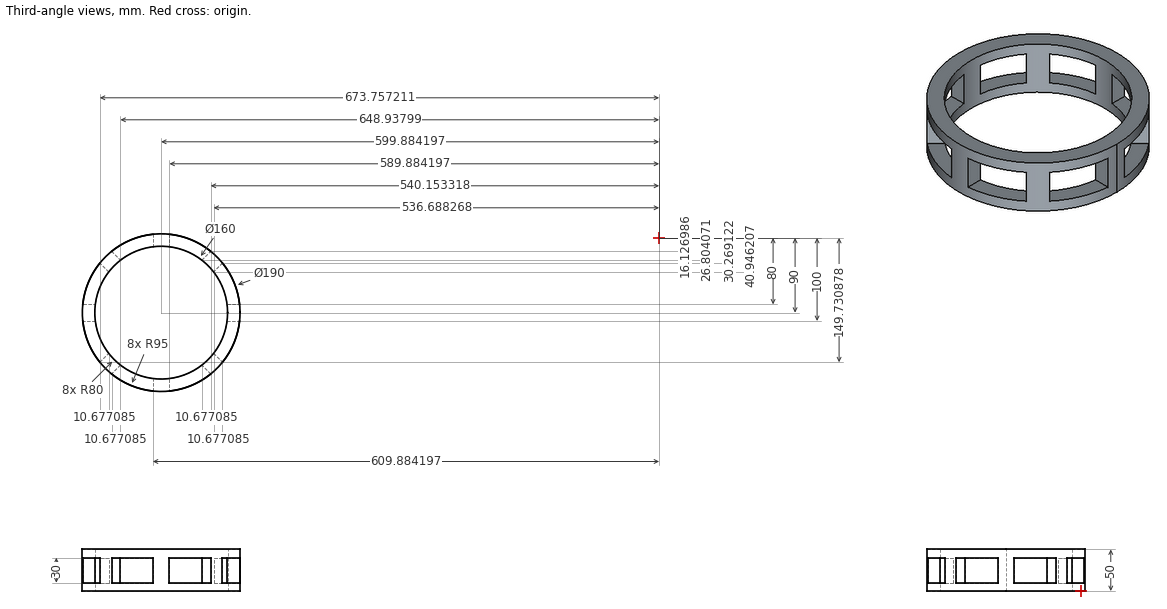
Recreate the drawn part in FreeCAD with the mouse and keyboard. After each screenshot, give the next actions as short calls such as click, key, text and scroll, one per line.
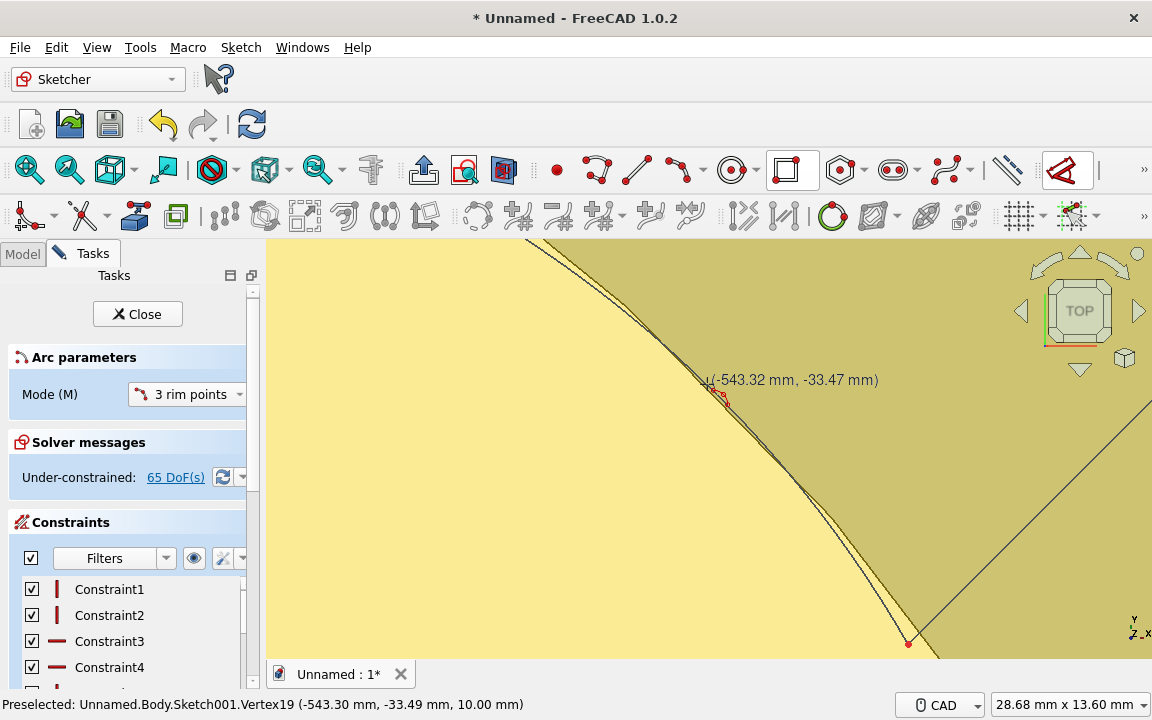
scroll(729, 361, down, 15)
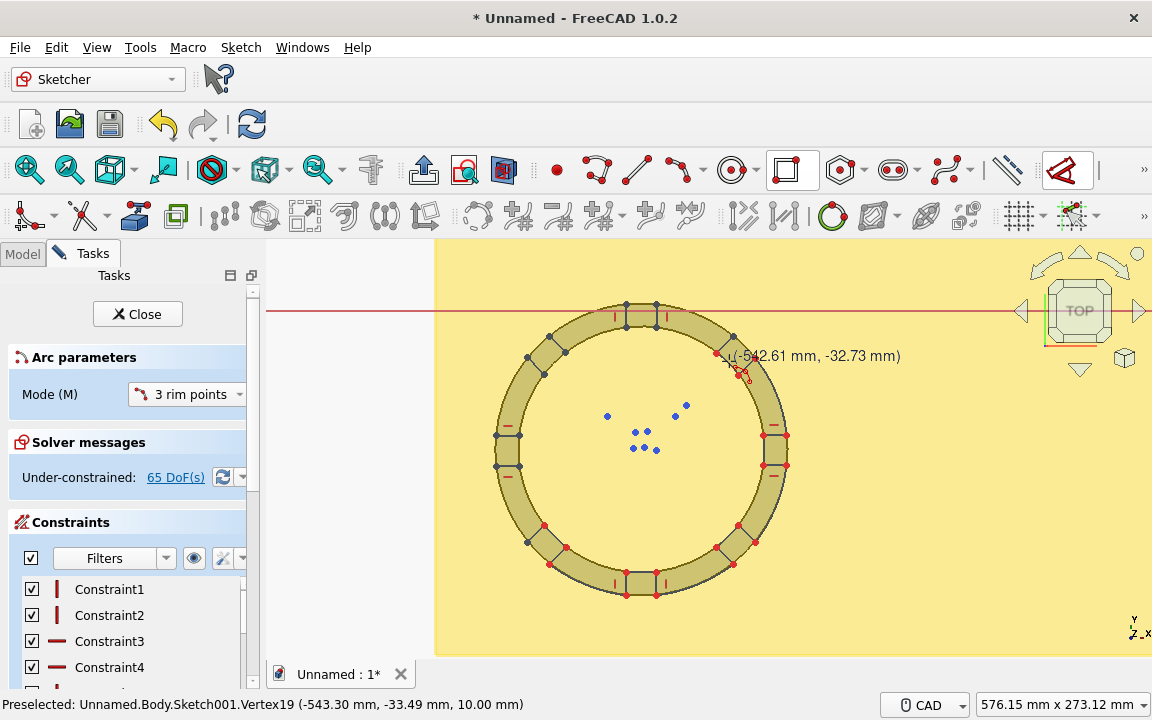
scroll(733, 336, up, 2)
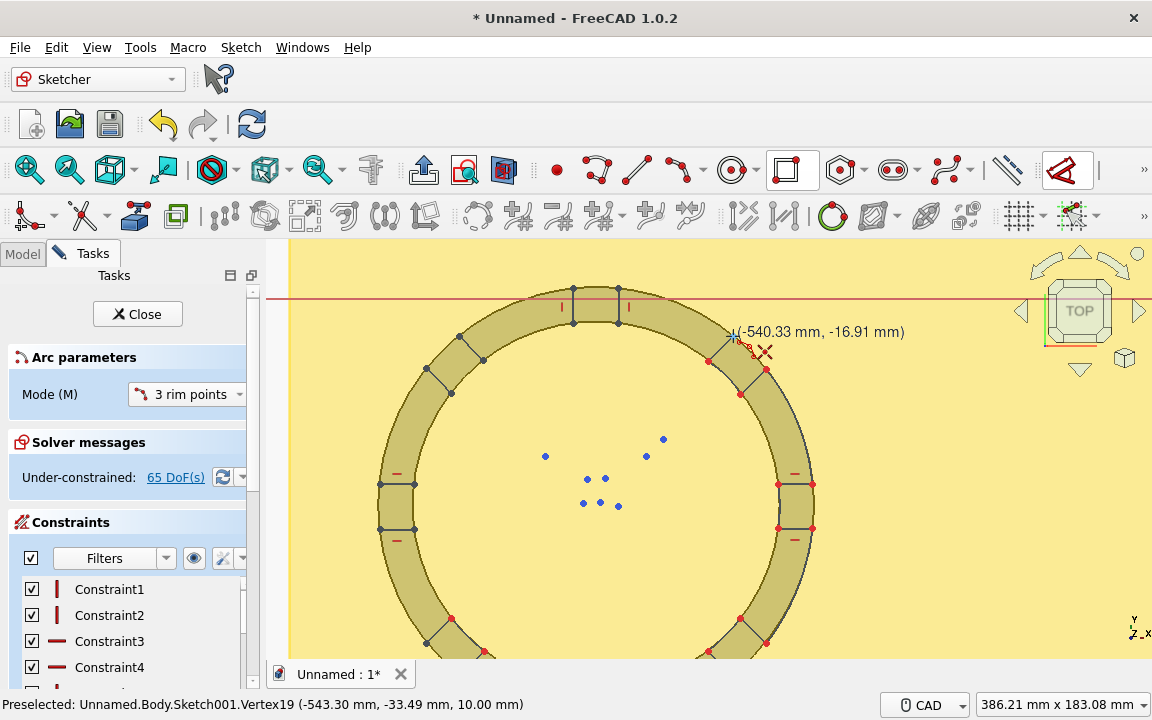
click(733, 336)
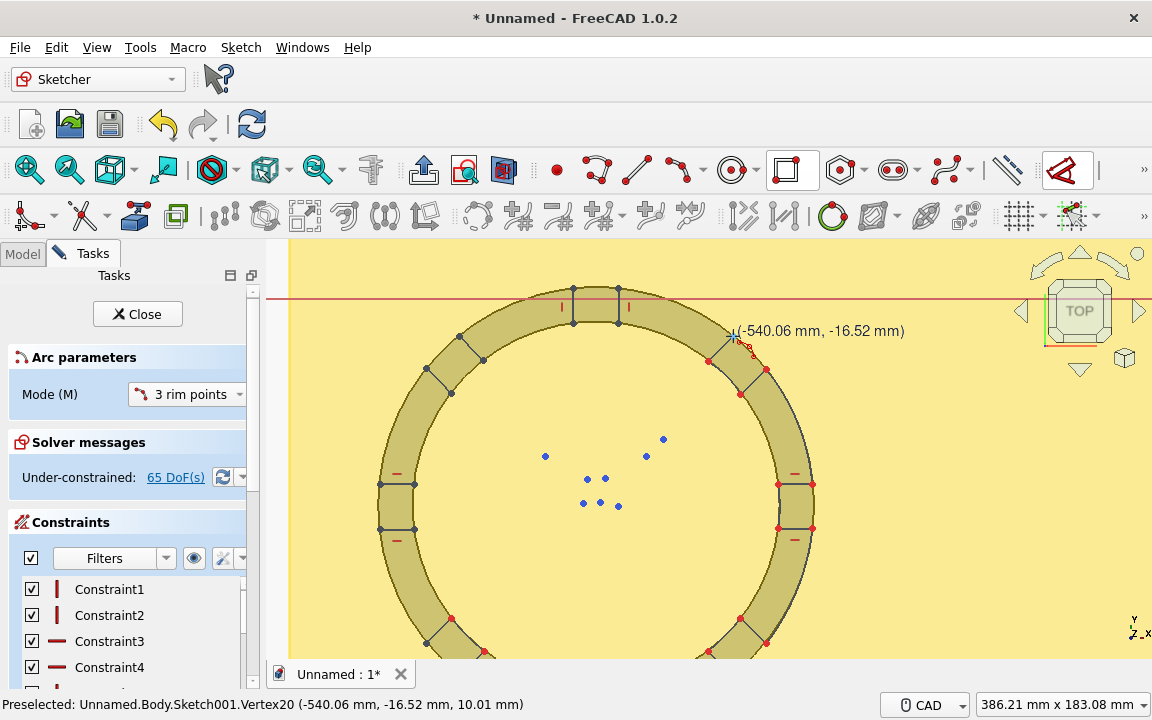
scroll(619, 288, up, 3)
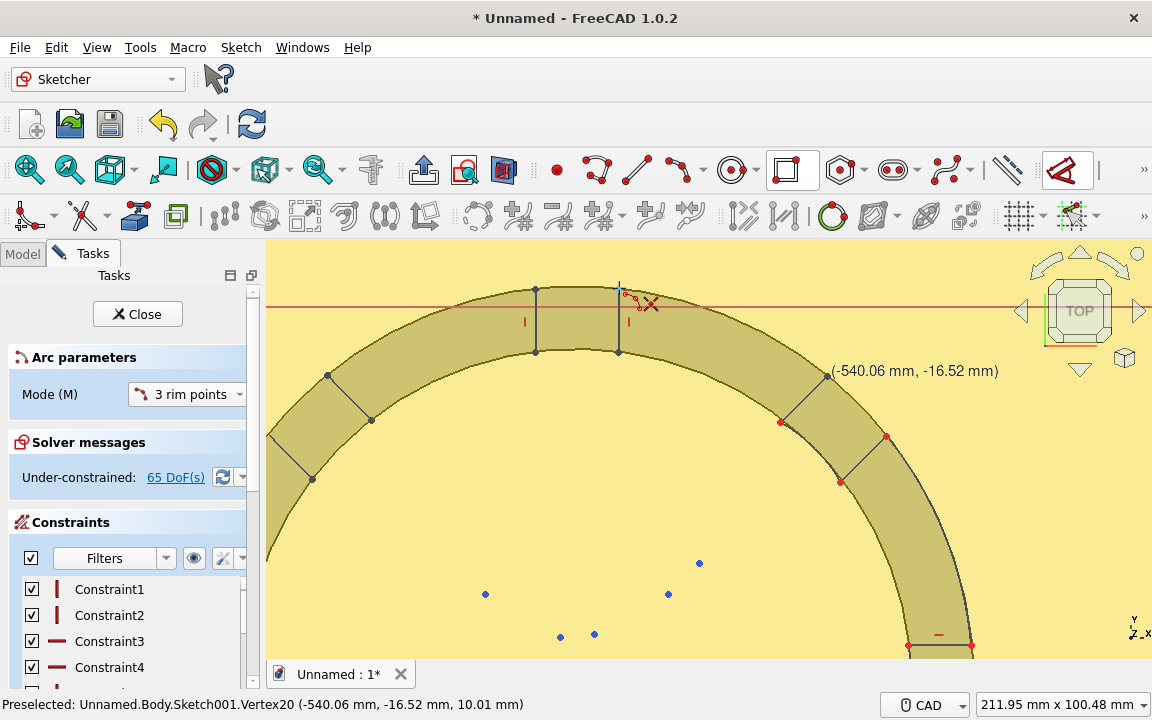
click(619, 290)
click(750, 326)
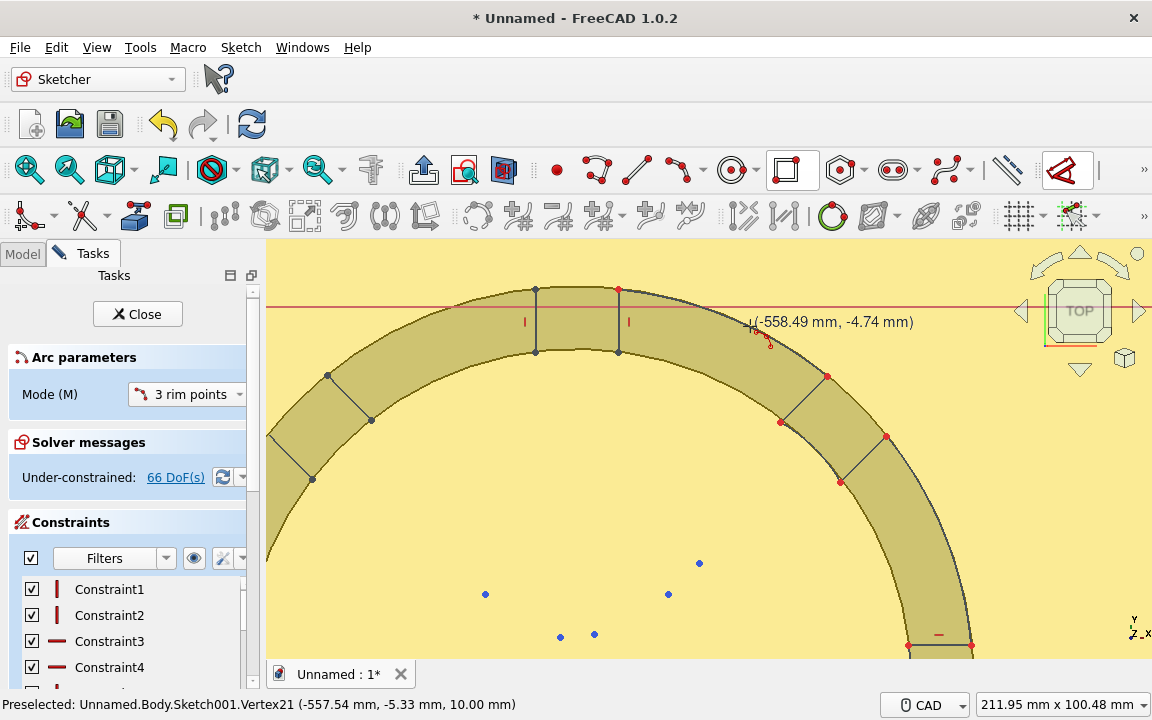
click(619, 353)
click(536, 353)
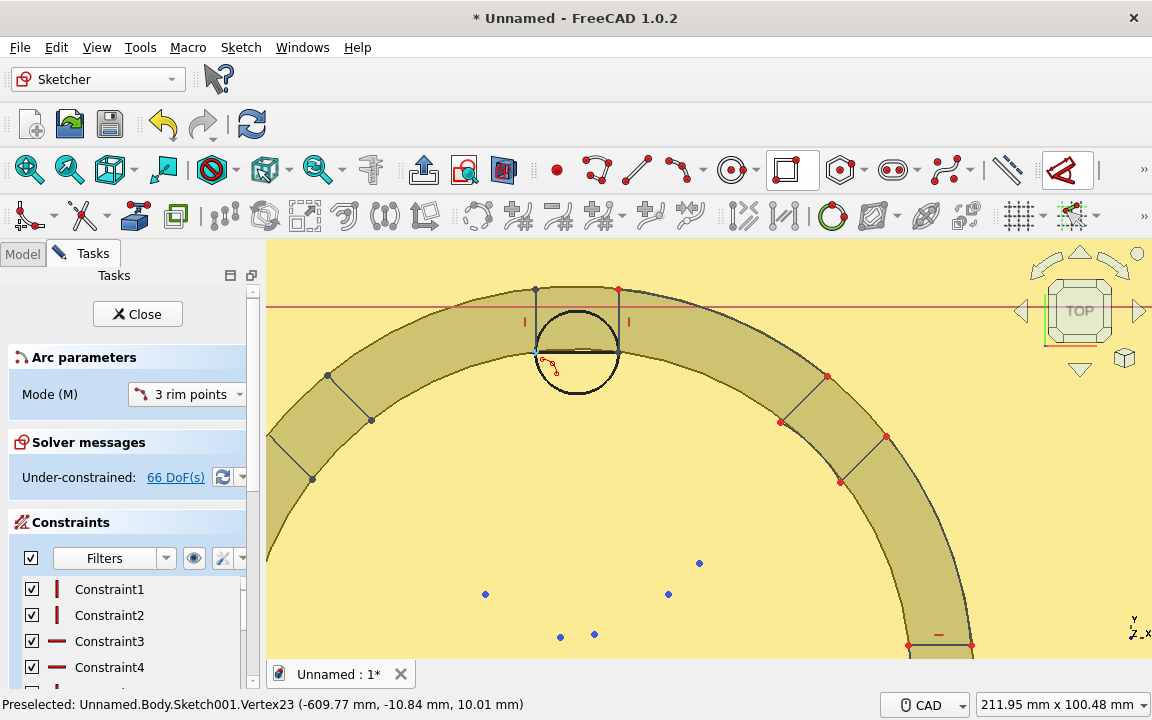
scroll(577, 349, up, 10)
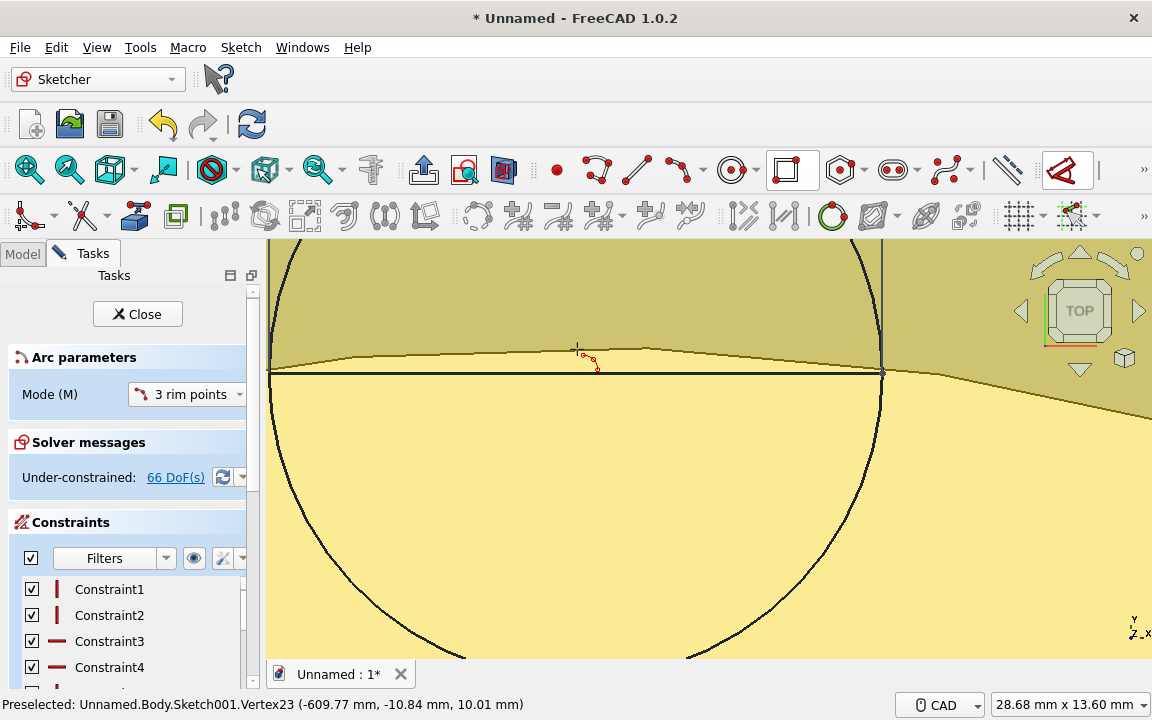
click(575, 347)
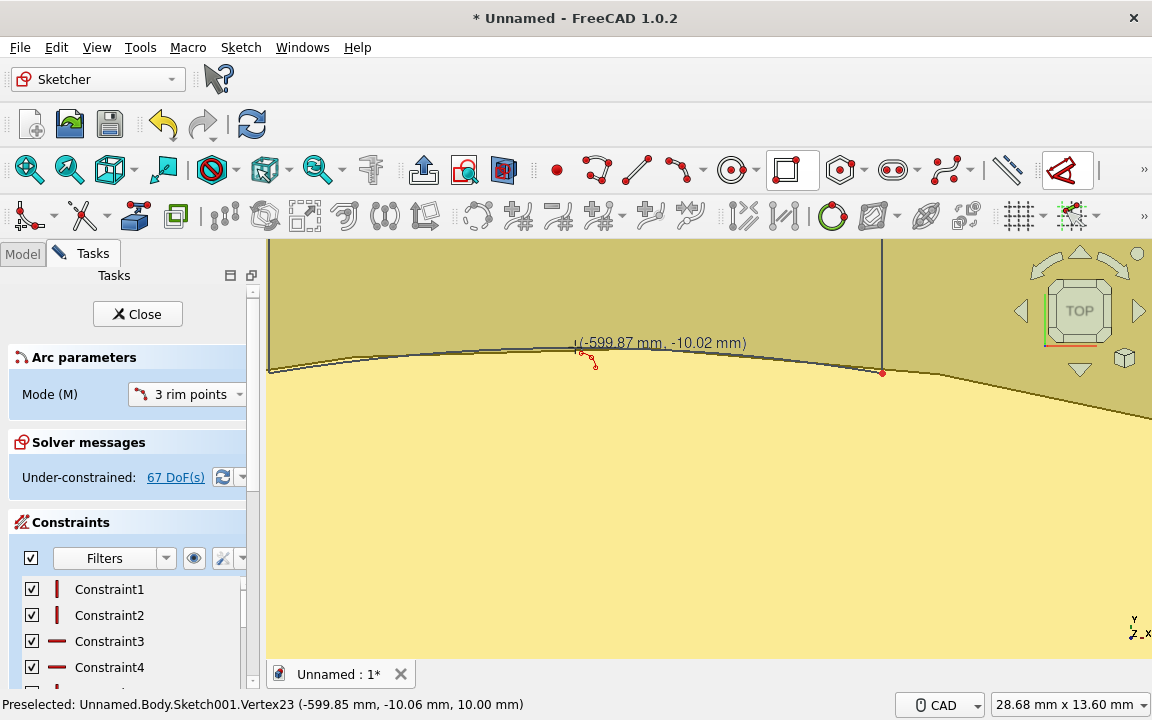
scroll(644, 325, down, 15)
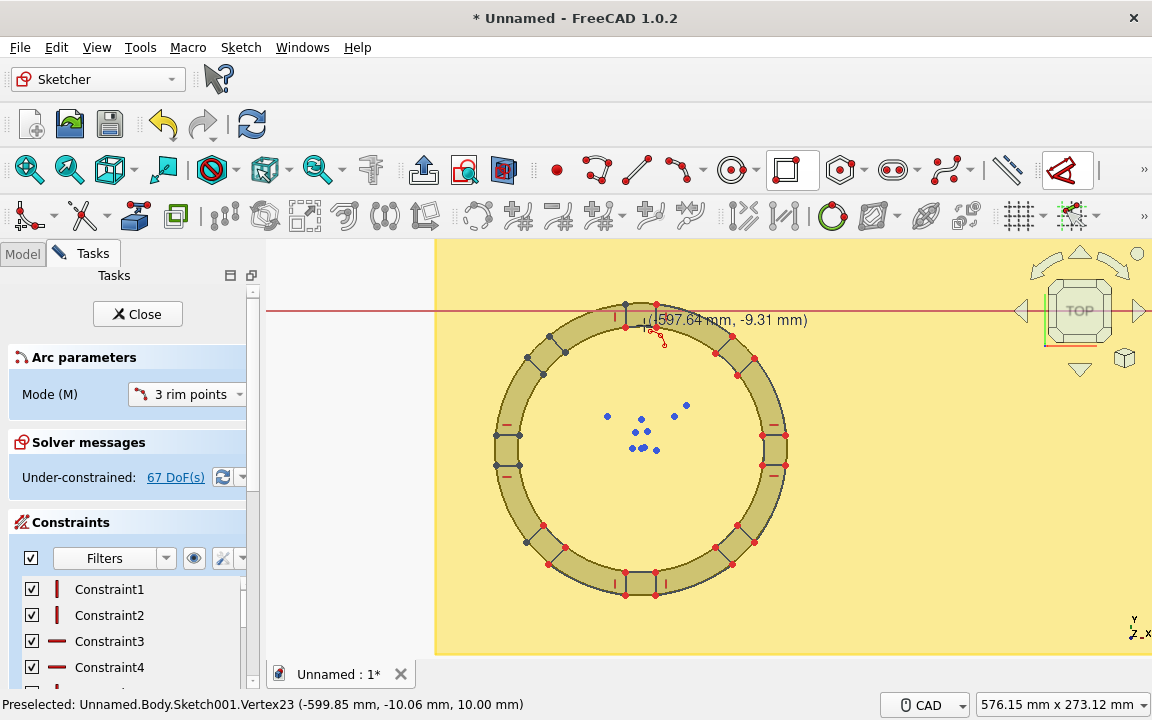
scroll(626, 304, up, 5)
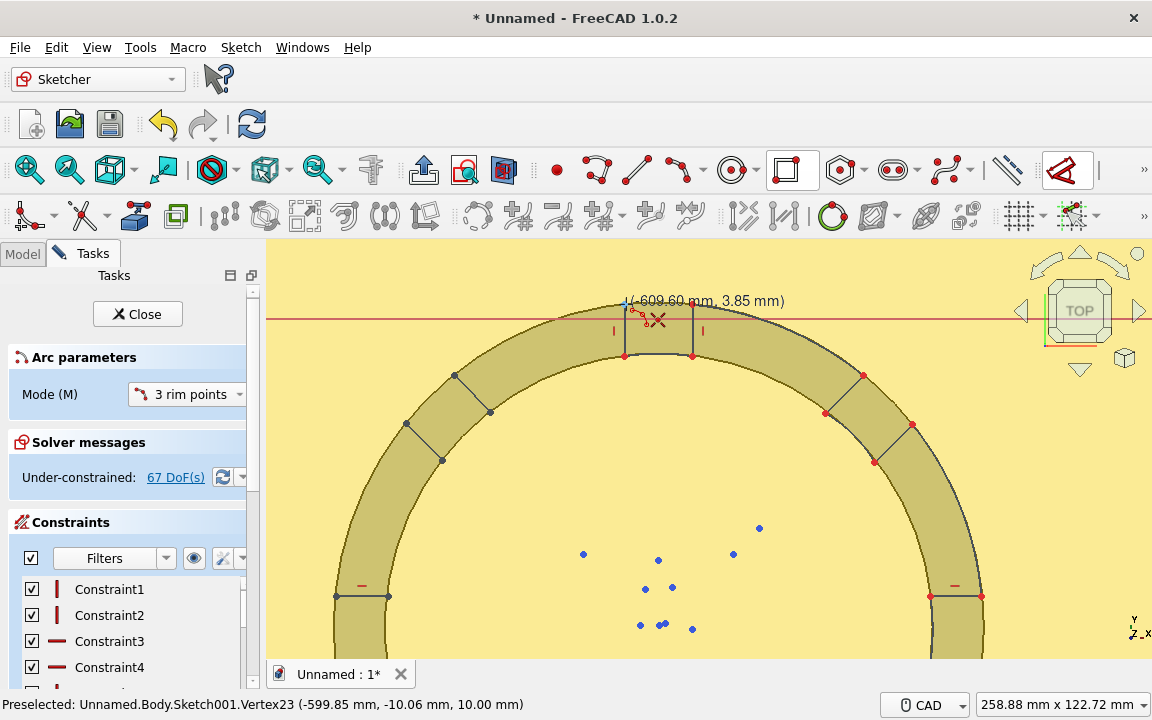
click(625, 305)
click(417, 391)
click(493, 341)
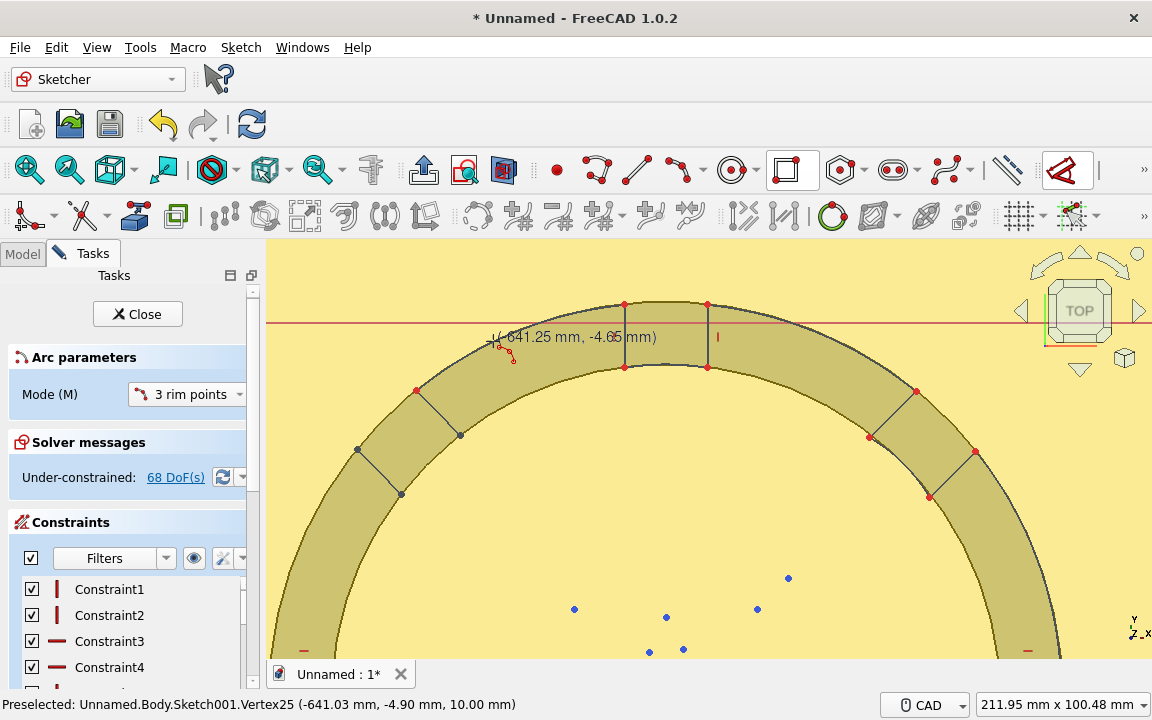
click(461, 436)
click(402, 495)